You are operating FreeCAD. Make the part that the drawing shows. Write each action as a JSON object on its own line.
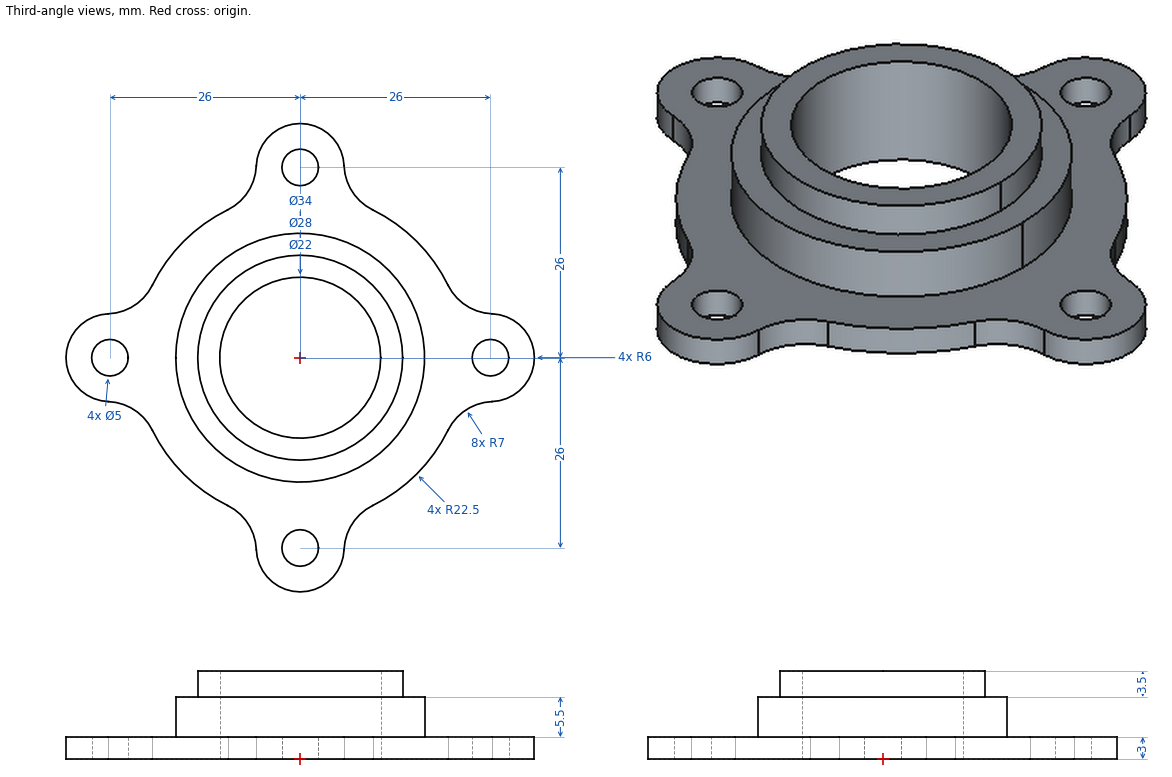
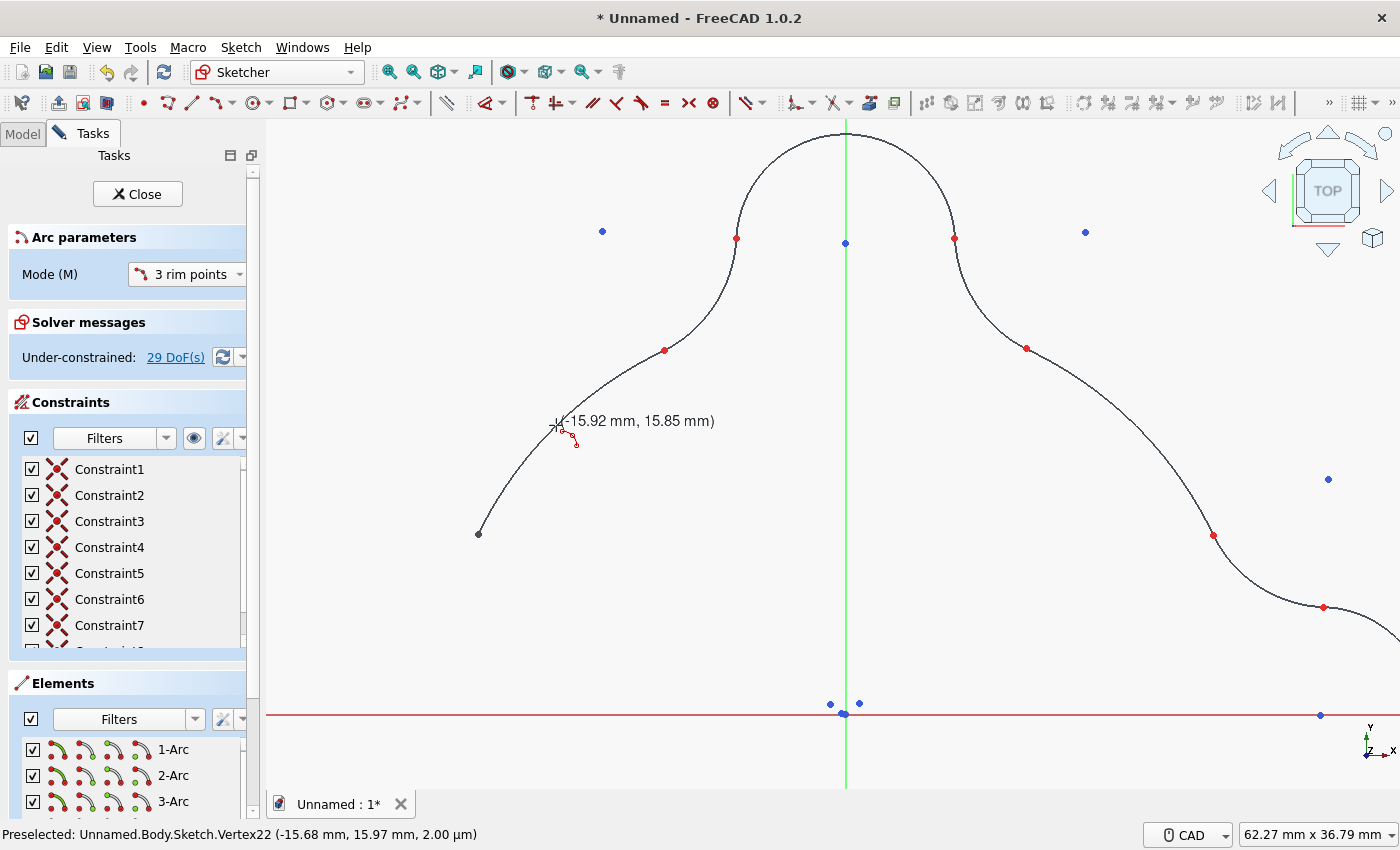
{"action": "left_click", "coordinate": [478, 535]}
{"action": "left_click", "coordinate": [368, 606]}
{"action": "left_click", "coordinate": [433, 585]}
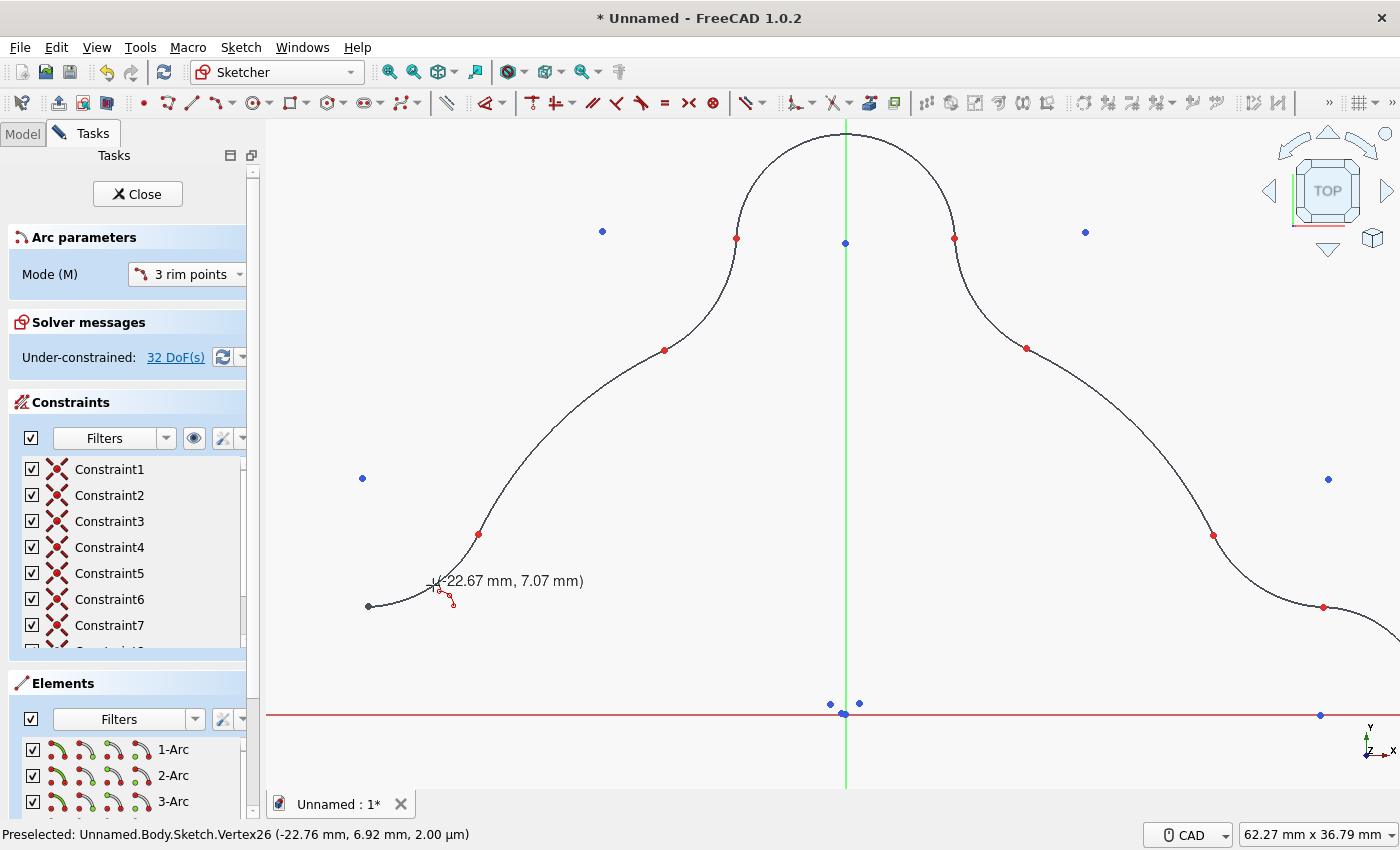
{"action": "left_click", "coordinate": [368, 607]}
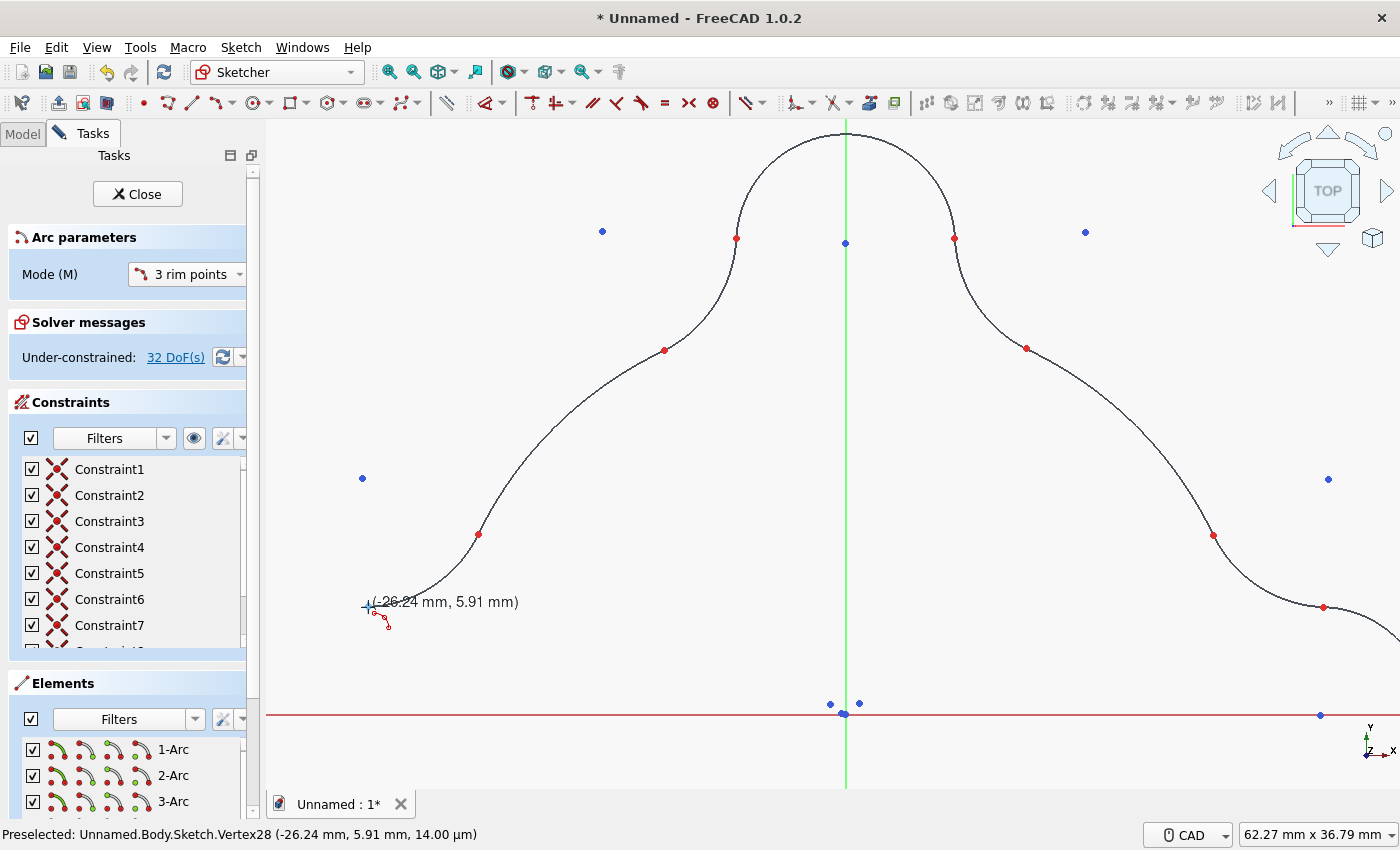
{"action": "scroll", "coordinate": [717, 302], "scroll_direction": "down", "scroll_amount": 5}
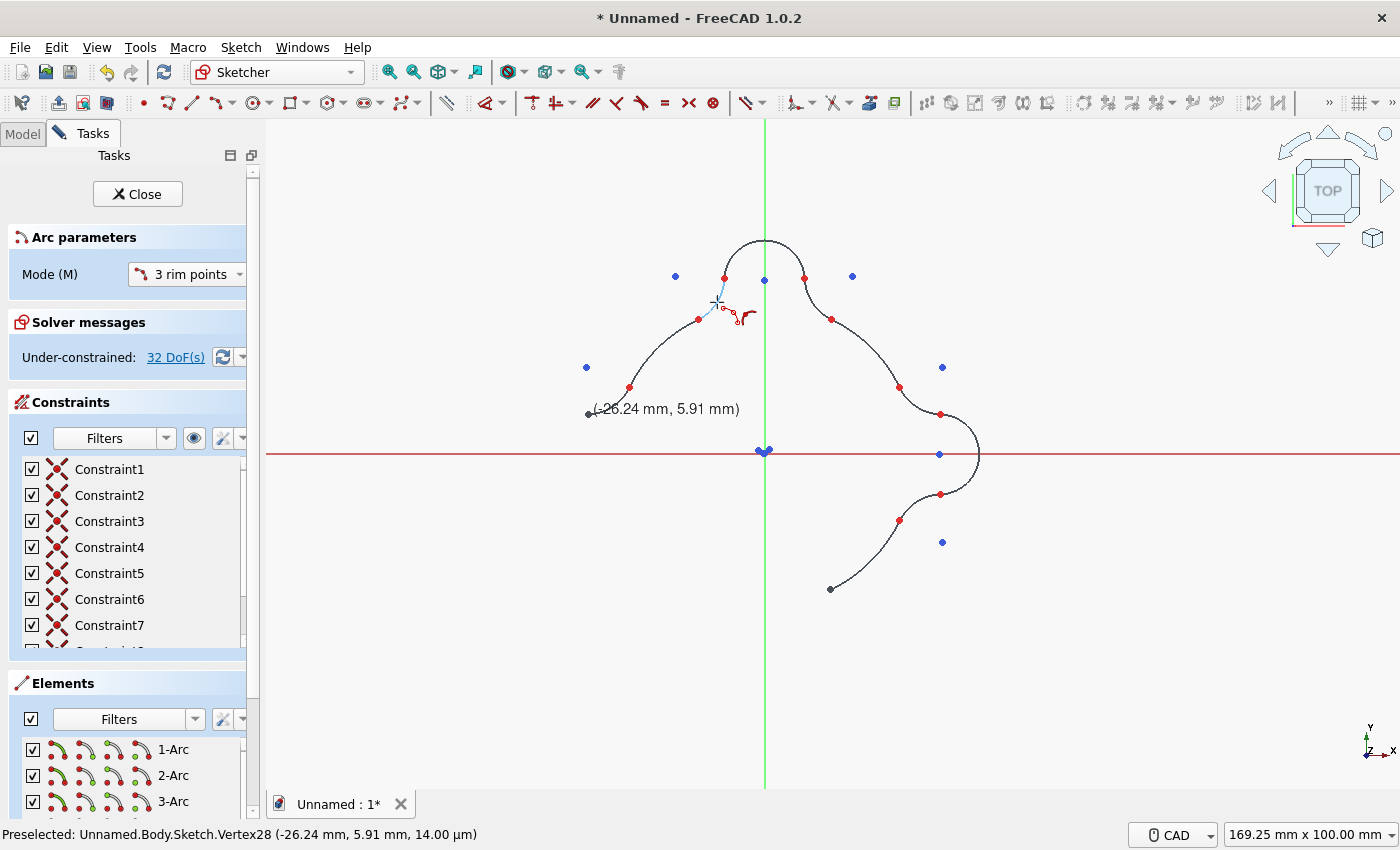
{"action": "left_click", "coordinate": [589, 494]}
{"action": "left_click", "coordinate": [558, 431]}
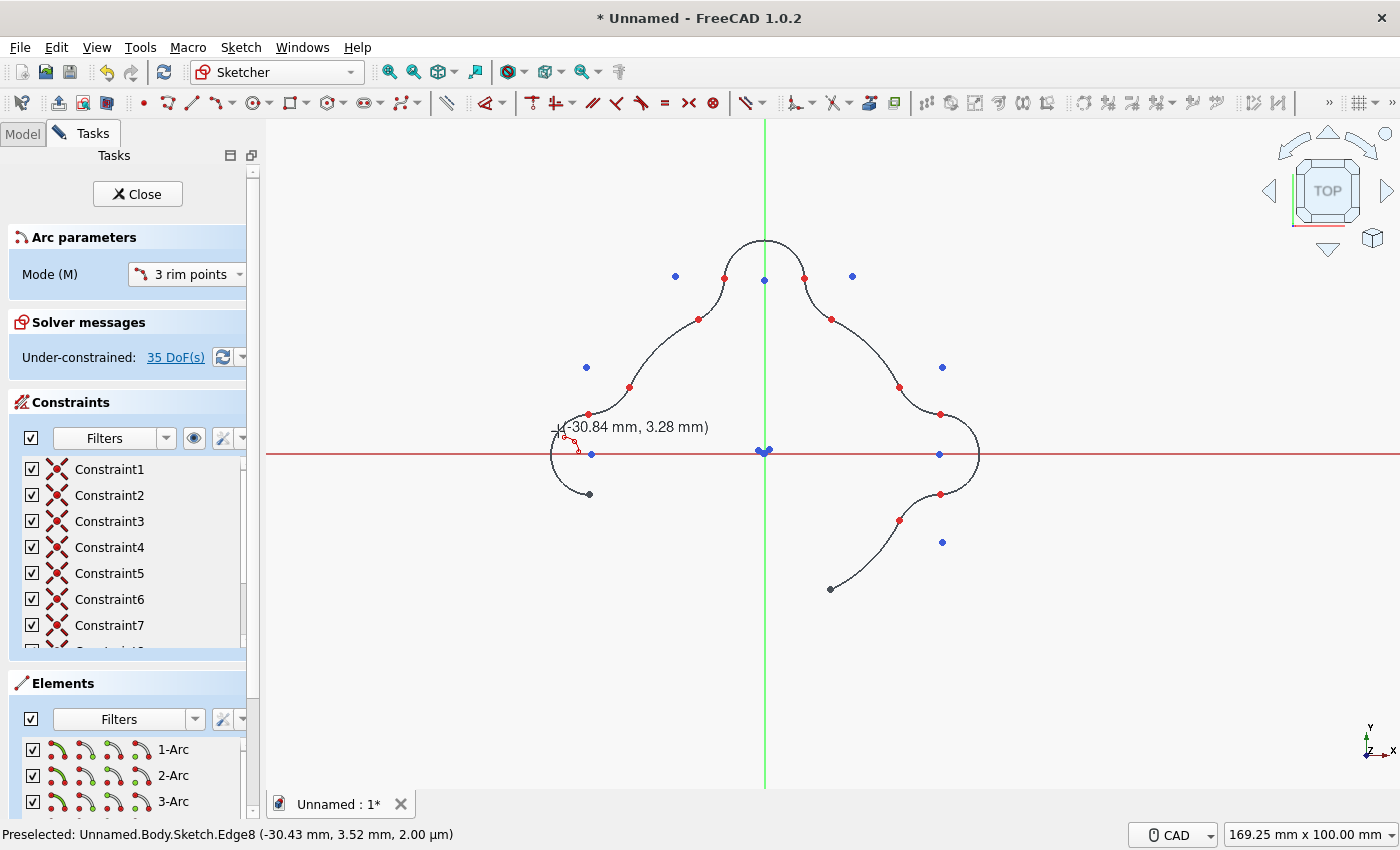
{"action": "left_click", "coordinate": [589, 495]}
{"action": "left_click", "coordinate": [629, 520]}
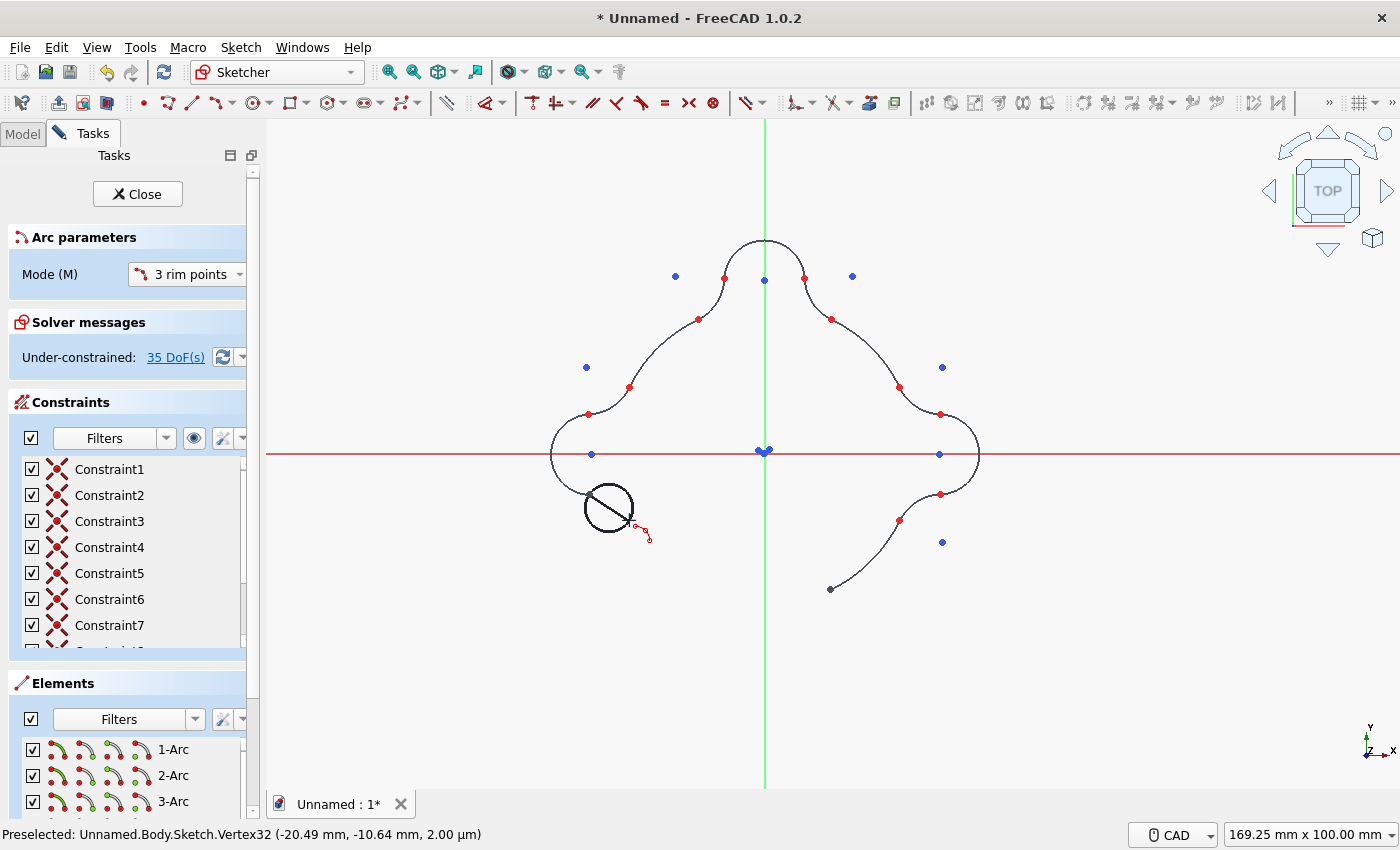
{"action": "scroll", "coordinate": [613, 502], "scroll_direction": "up", "scroll_amount": 5}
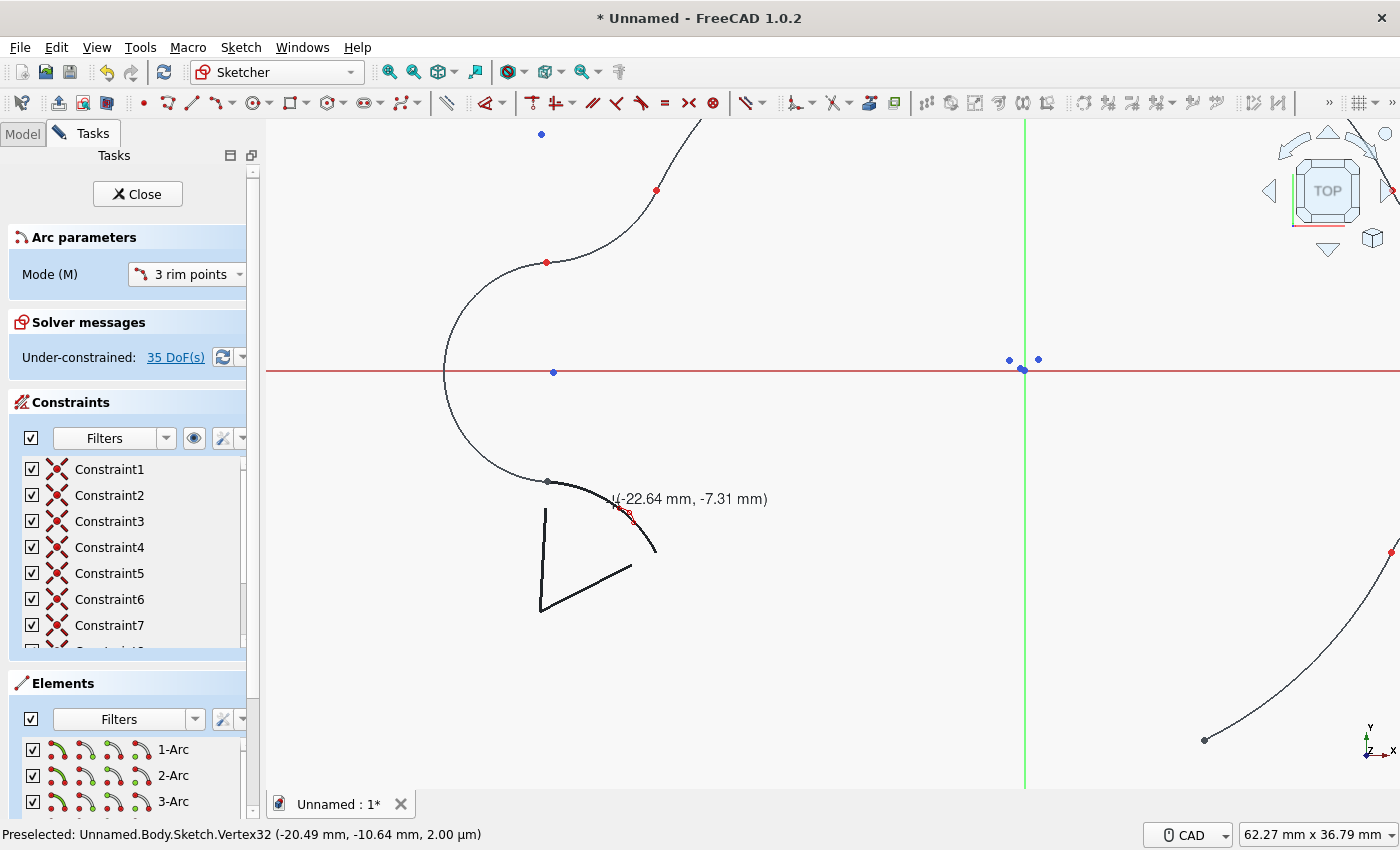
{"action": "left_click", "coordinate": [612, 500]}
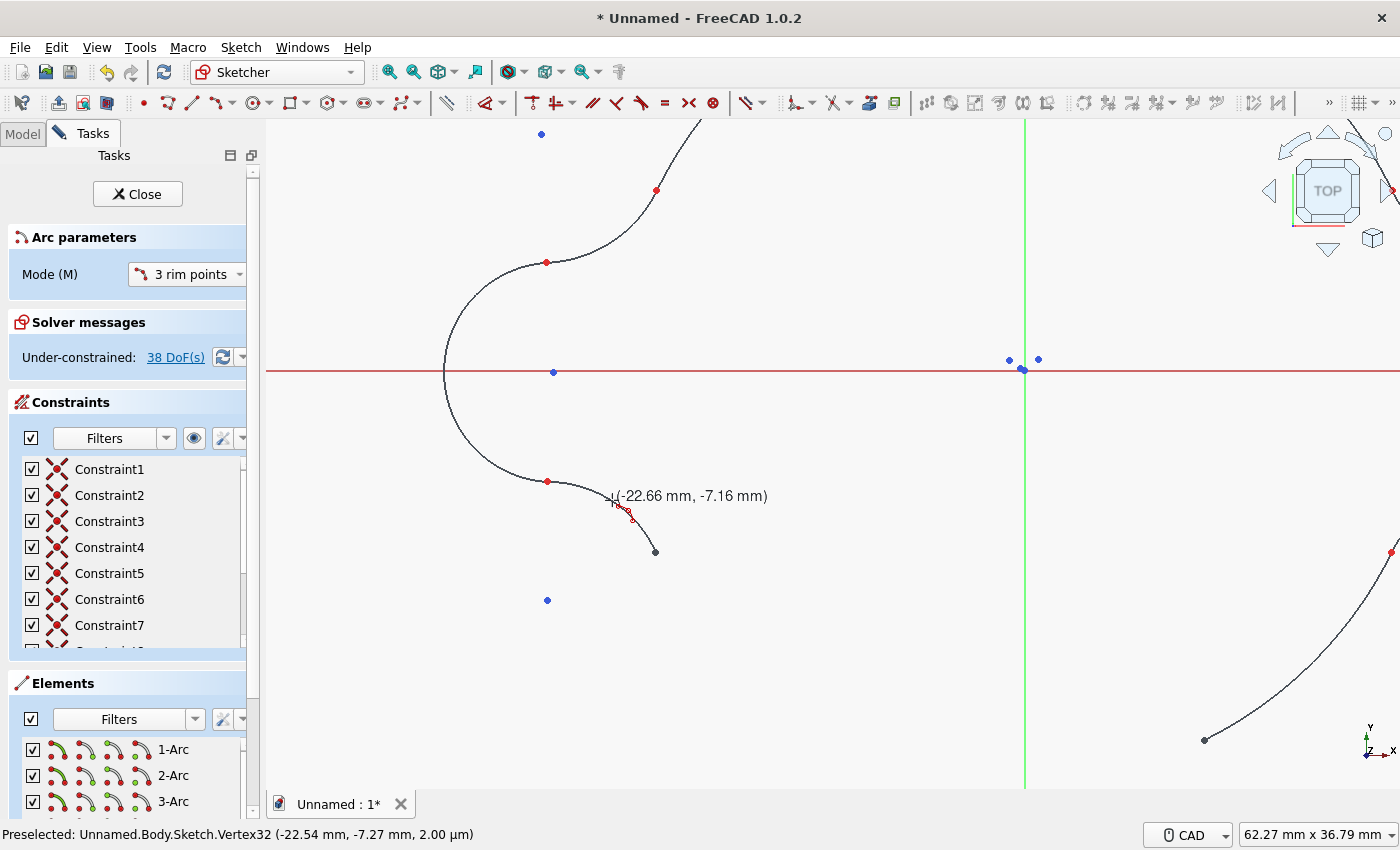
{"action": "left_click", "coordinate": [656, 553]}
{"action": "left_click", "coordinate": [844, 738]}
{"action": "left_click", "coordinate": [735, 660]}